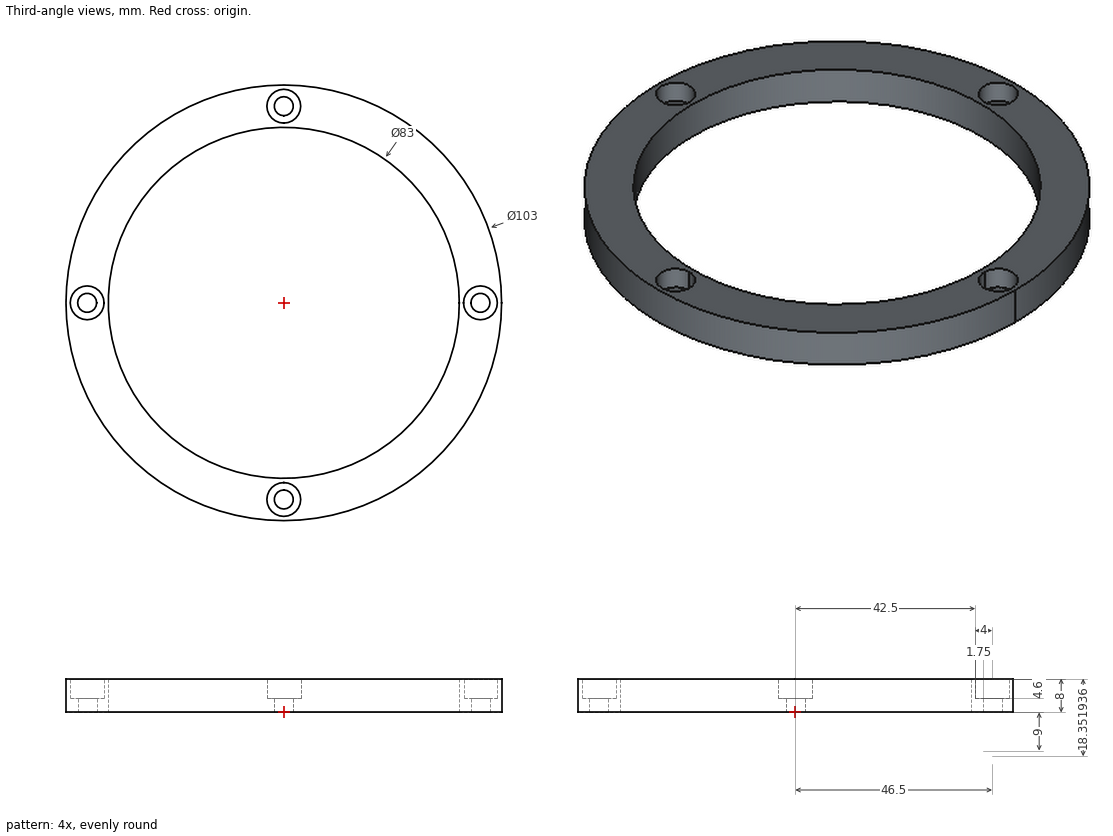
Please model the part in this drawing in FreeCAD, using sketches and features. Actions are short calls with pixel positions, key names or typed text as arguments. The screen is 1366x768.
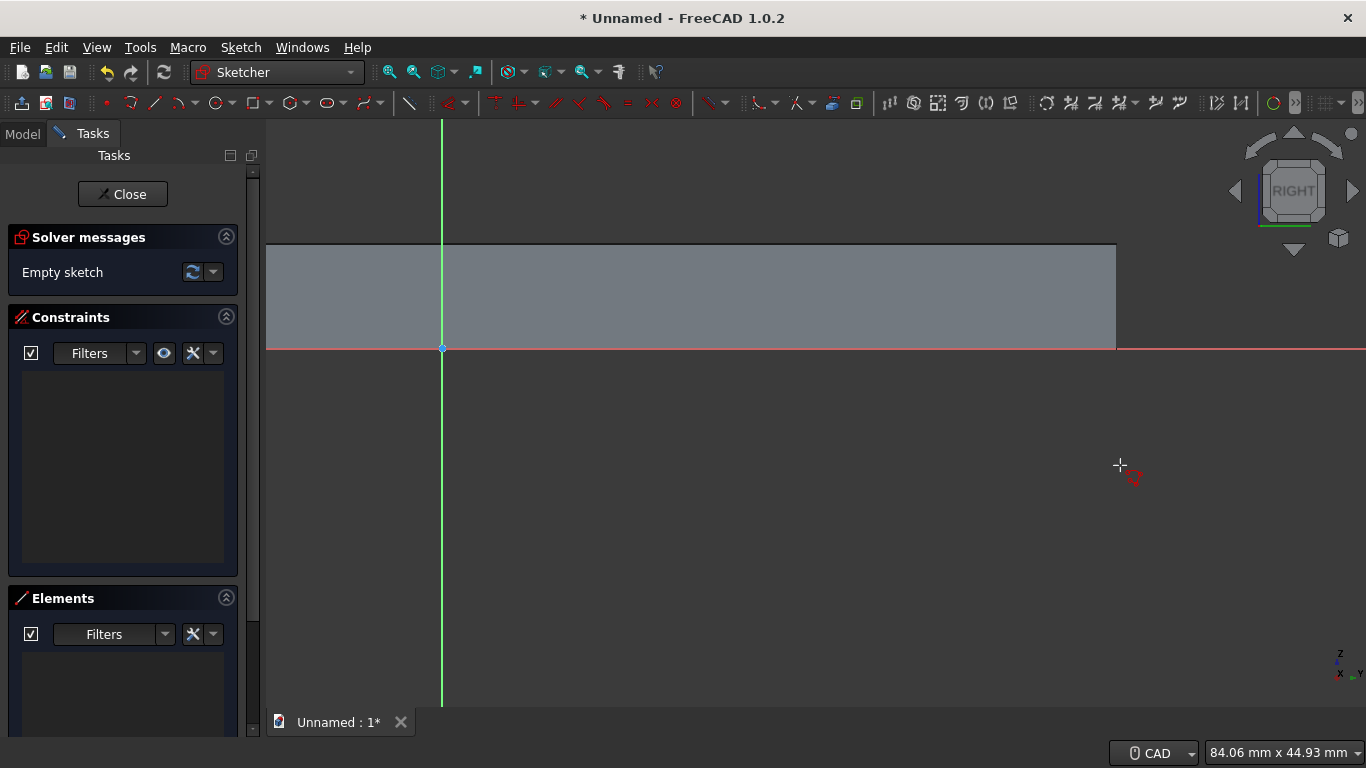
click(999, 304)
click(1022, 304)
click(1022, 466)
click(1051, 484)
click(1051, 244)
click(999, 244)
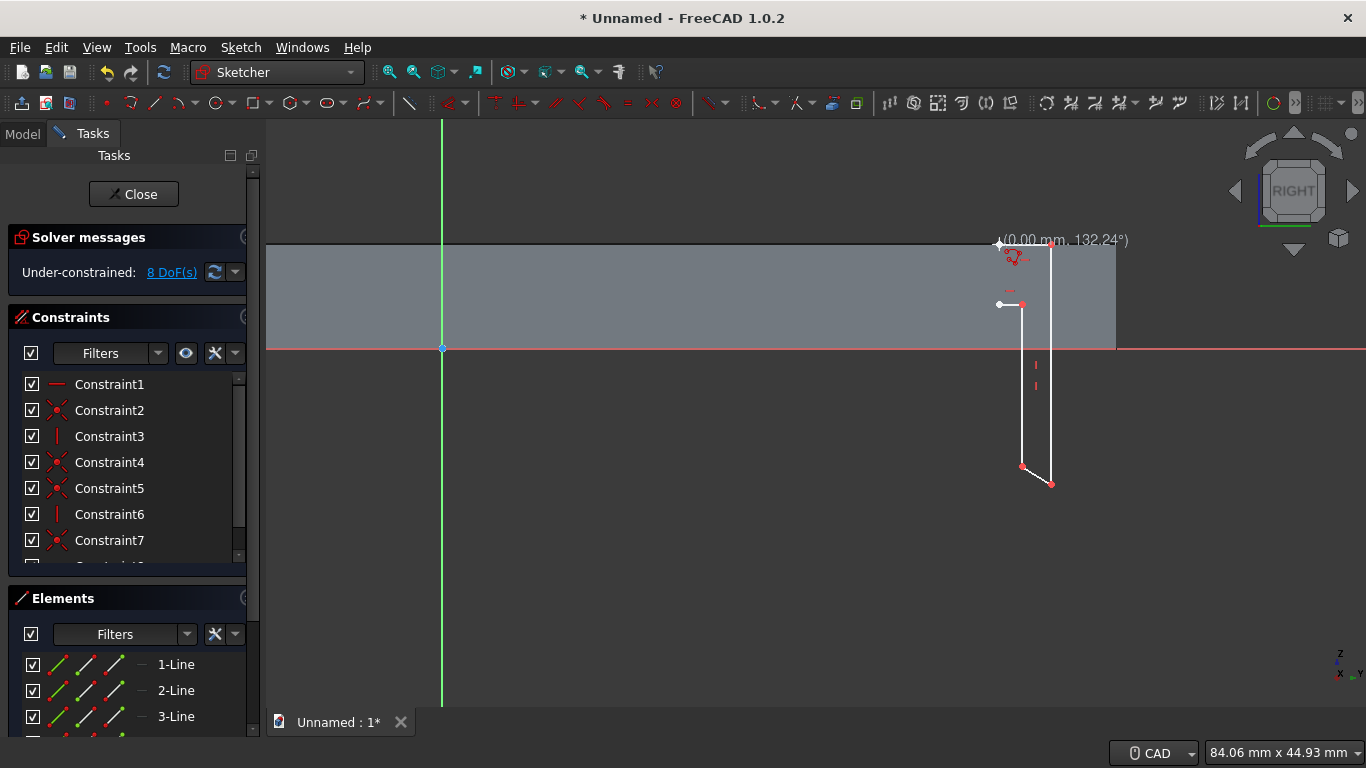
scroll(999, 304, up, 2)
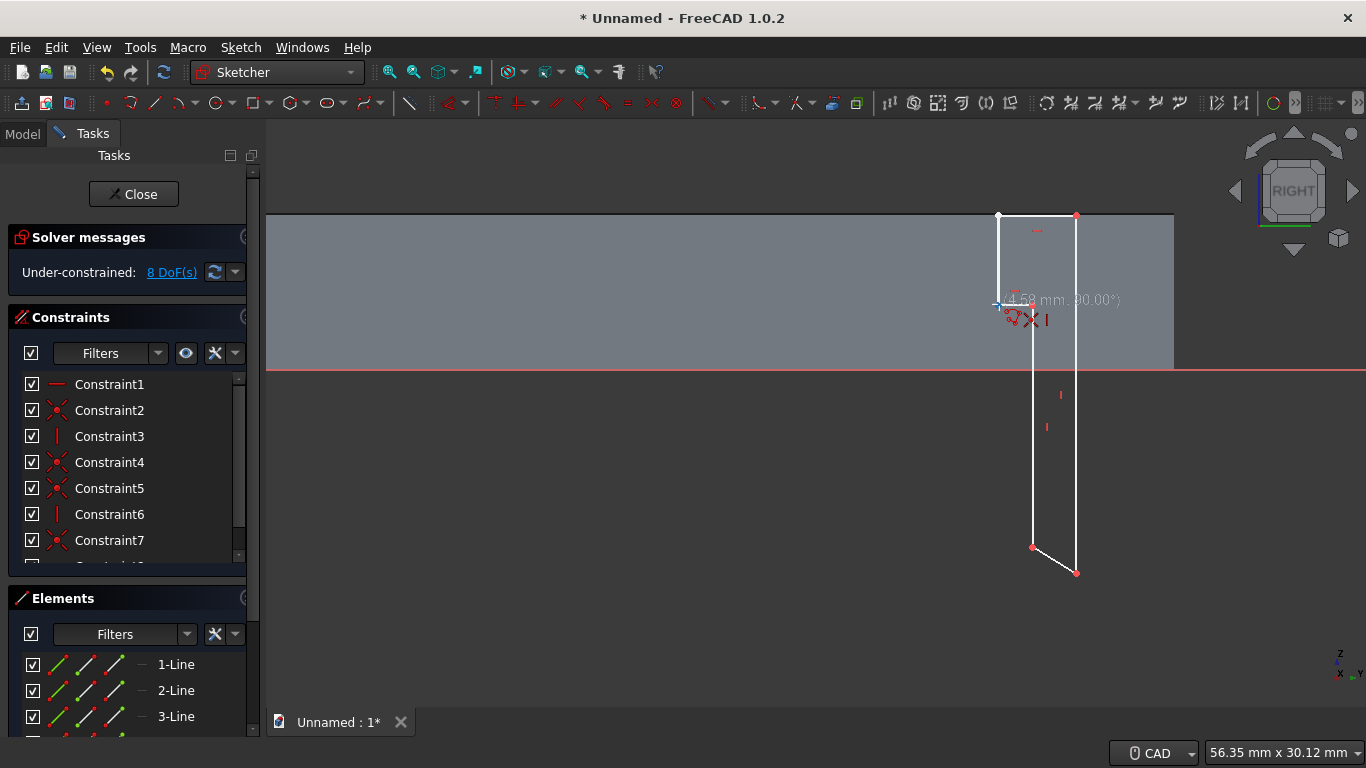
click(999, 305)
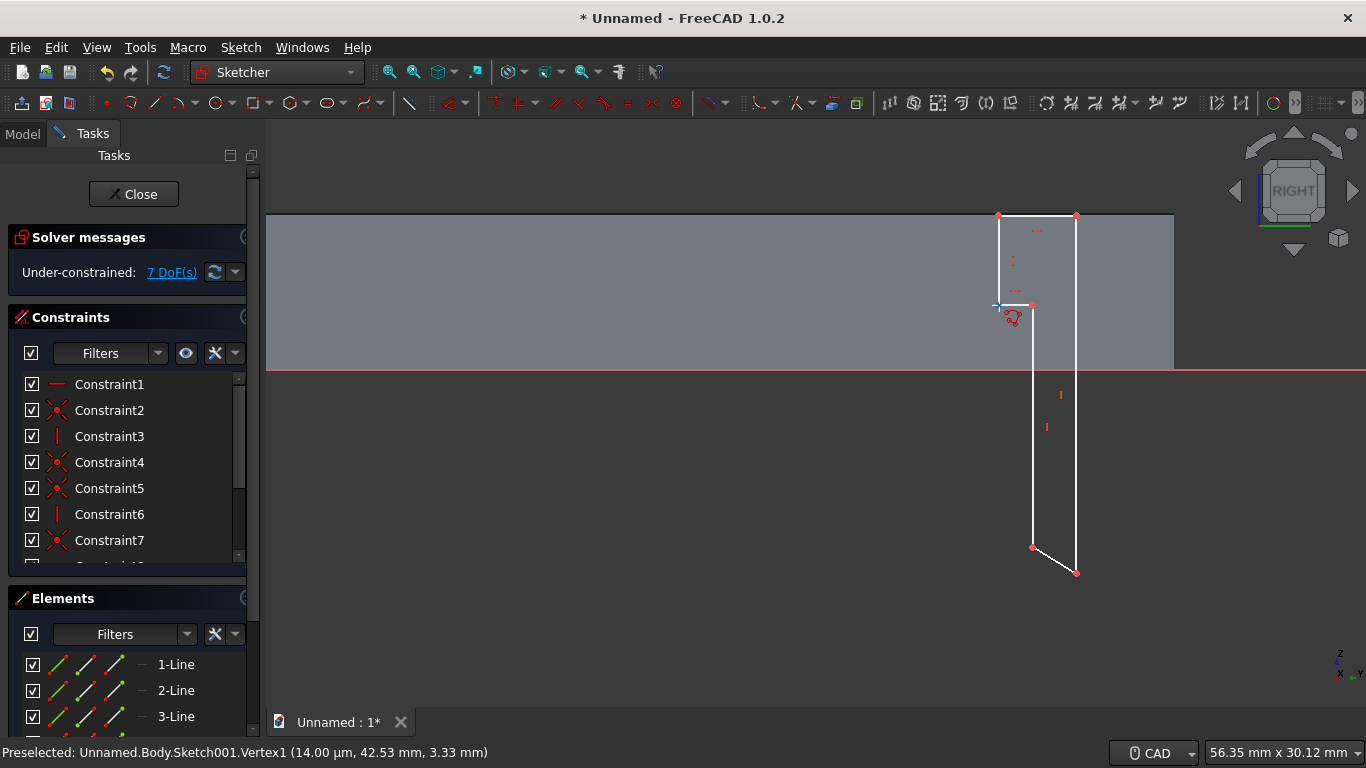
click(156, 104)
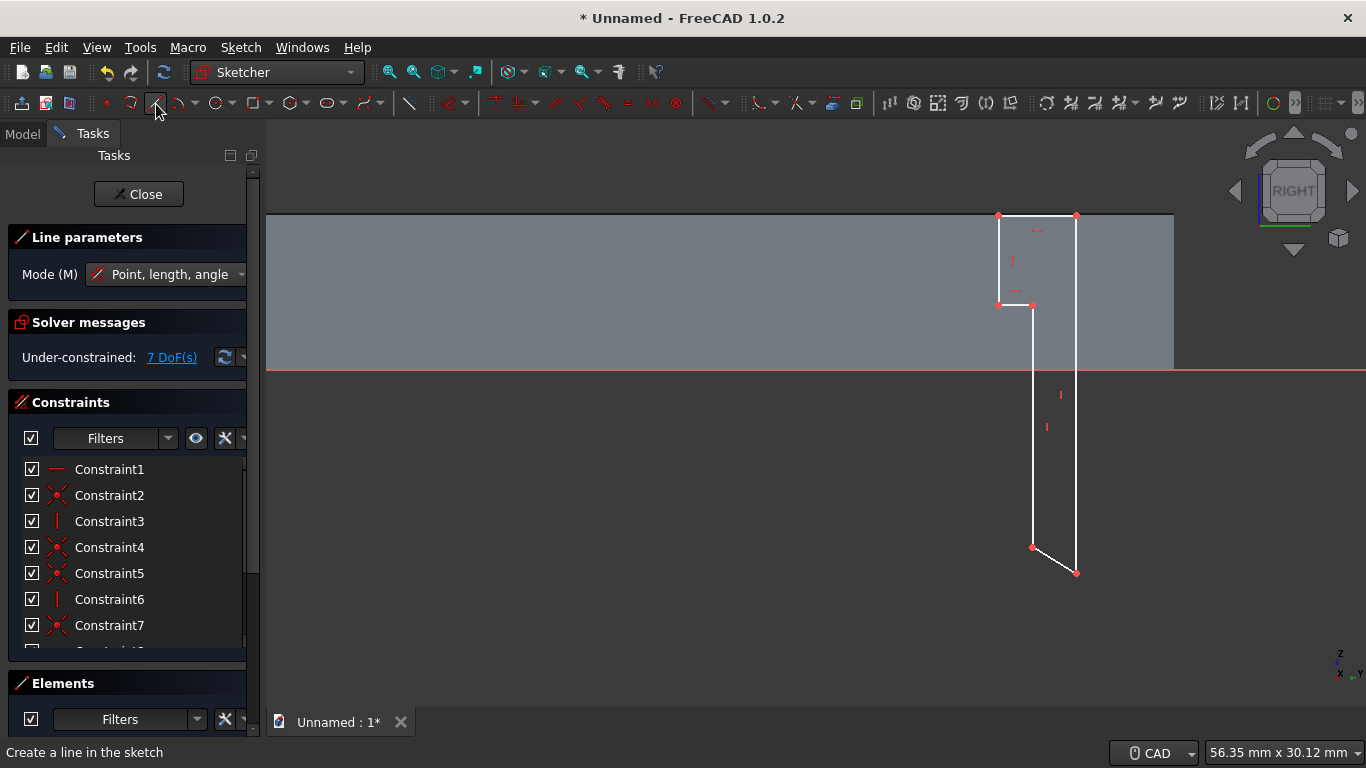
click(1076, 608)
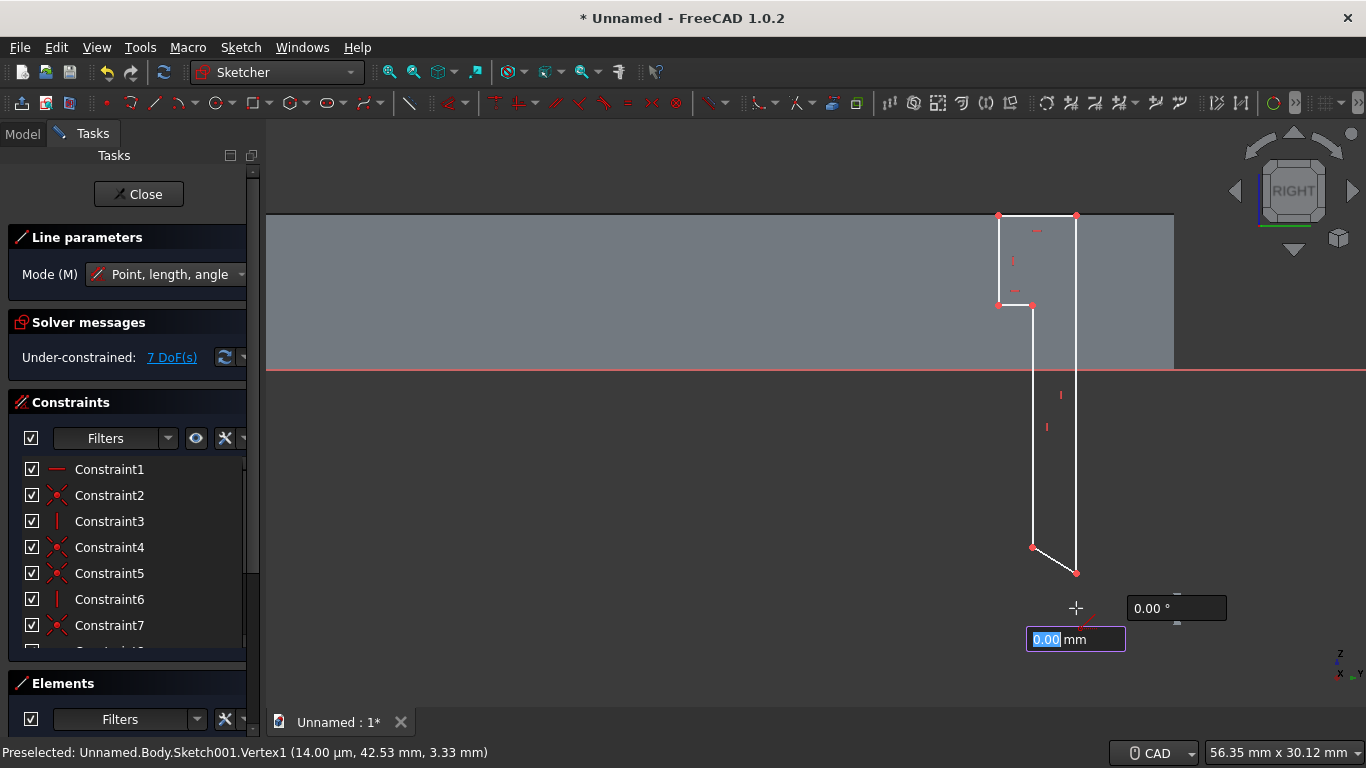
scroll(1002, 307, down, 2)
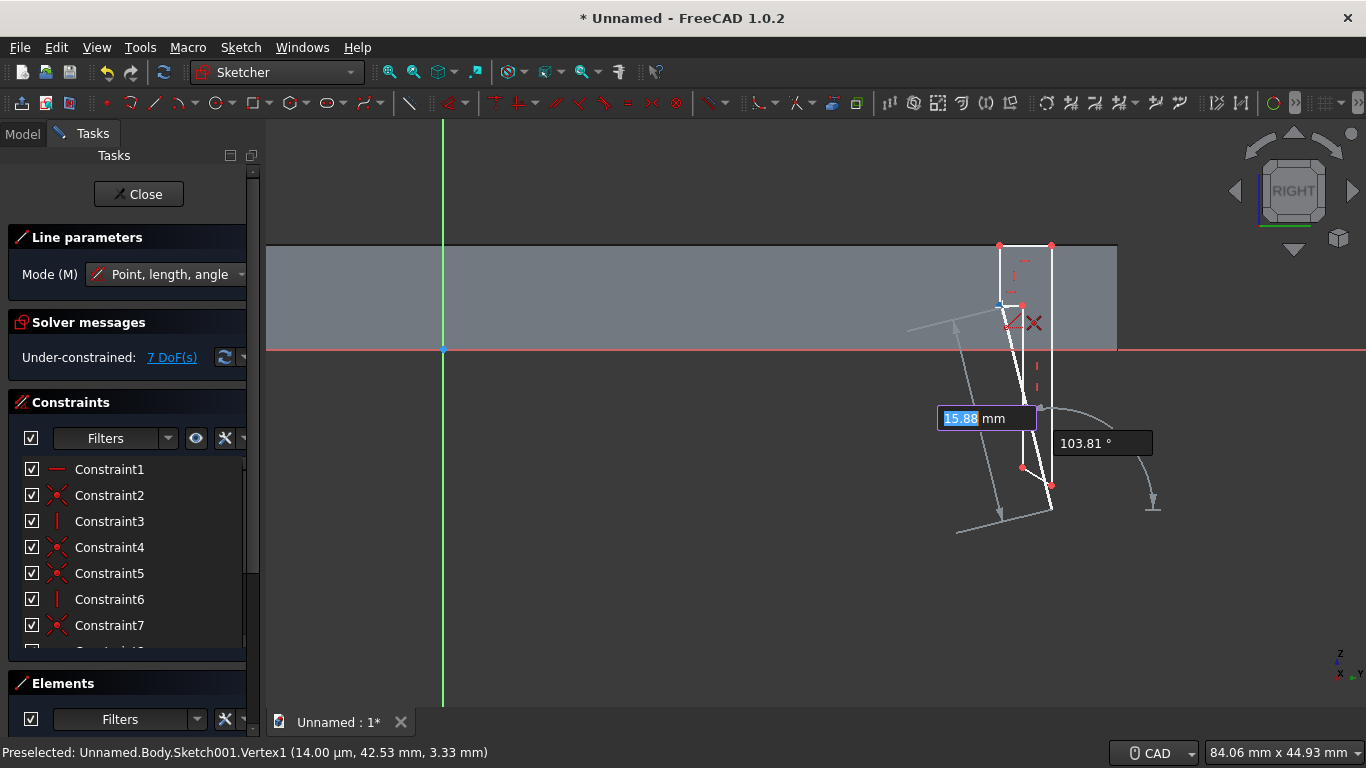
click(1052, 581)
key(Escape)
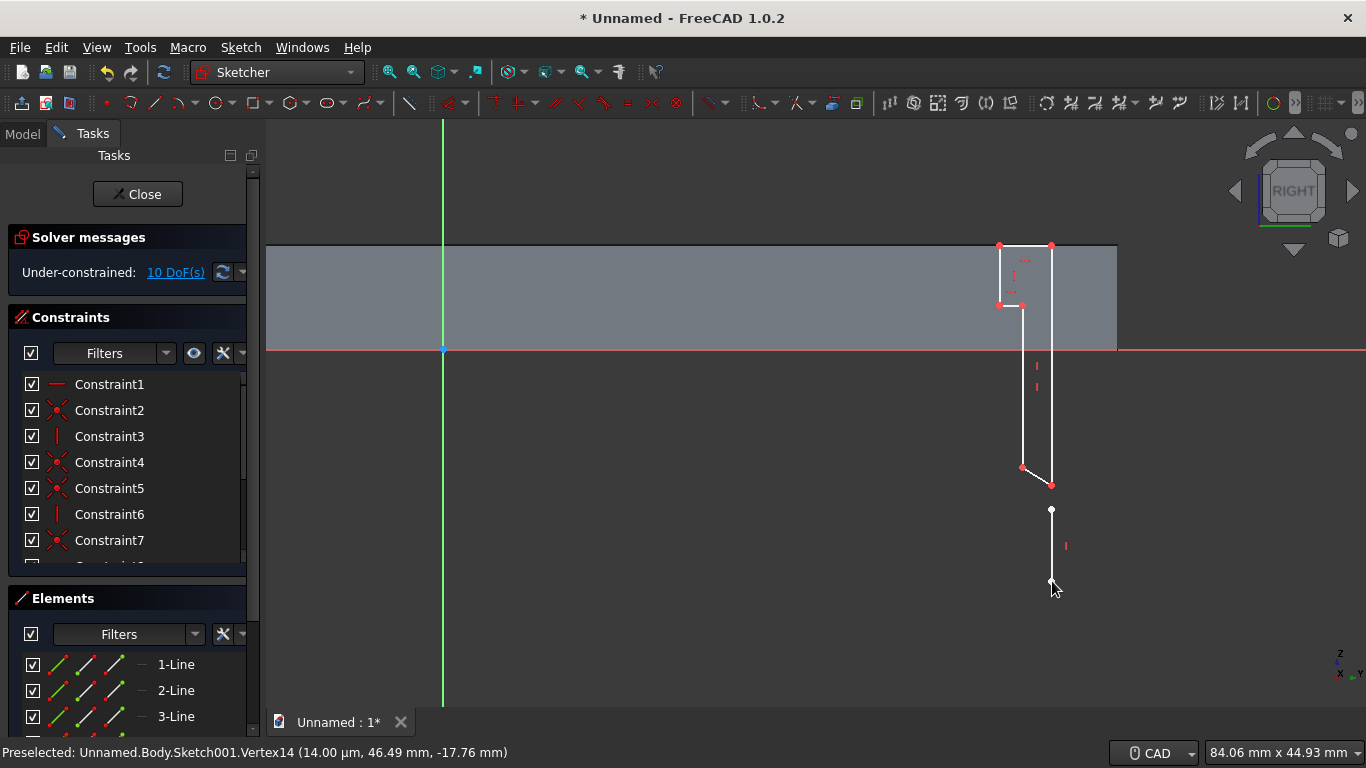
click(1052, 531)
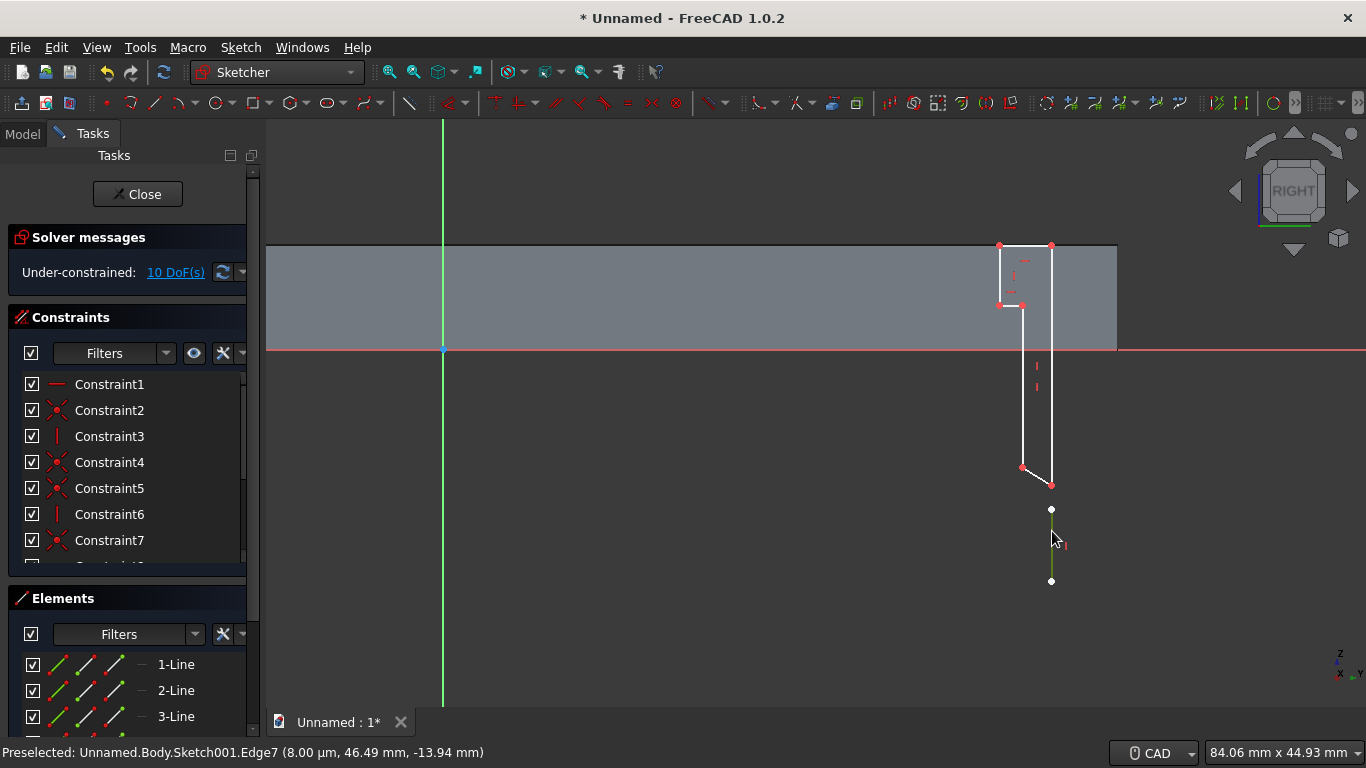
click(410, 104)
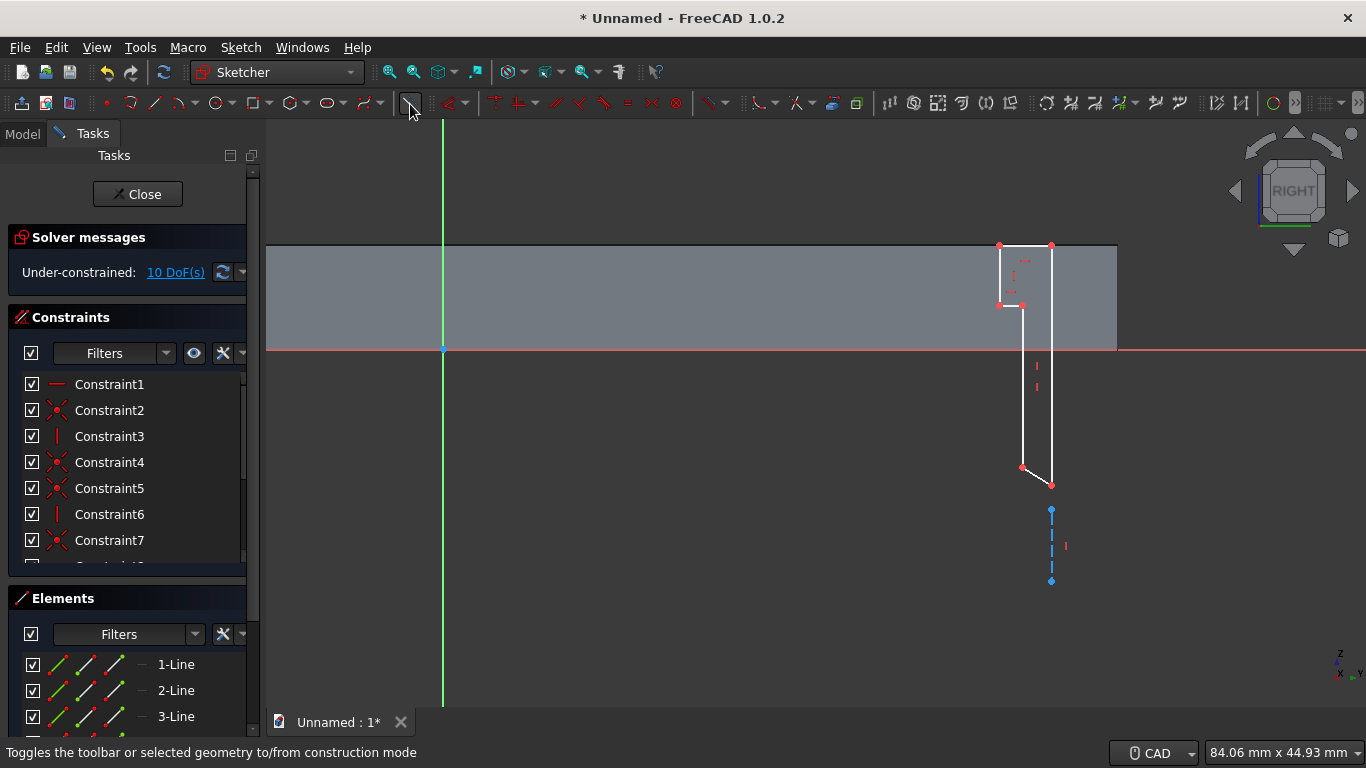
click(1036, 246)